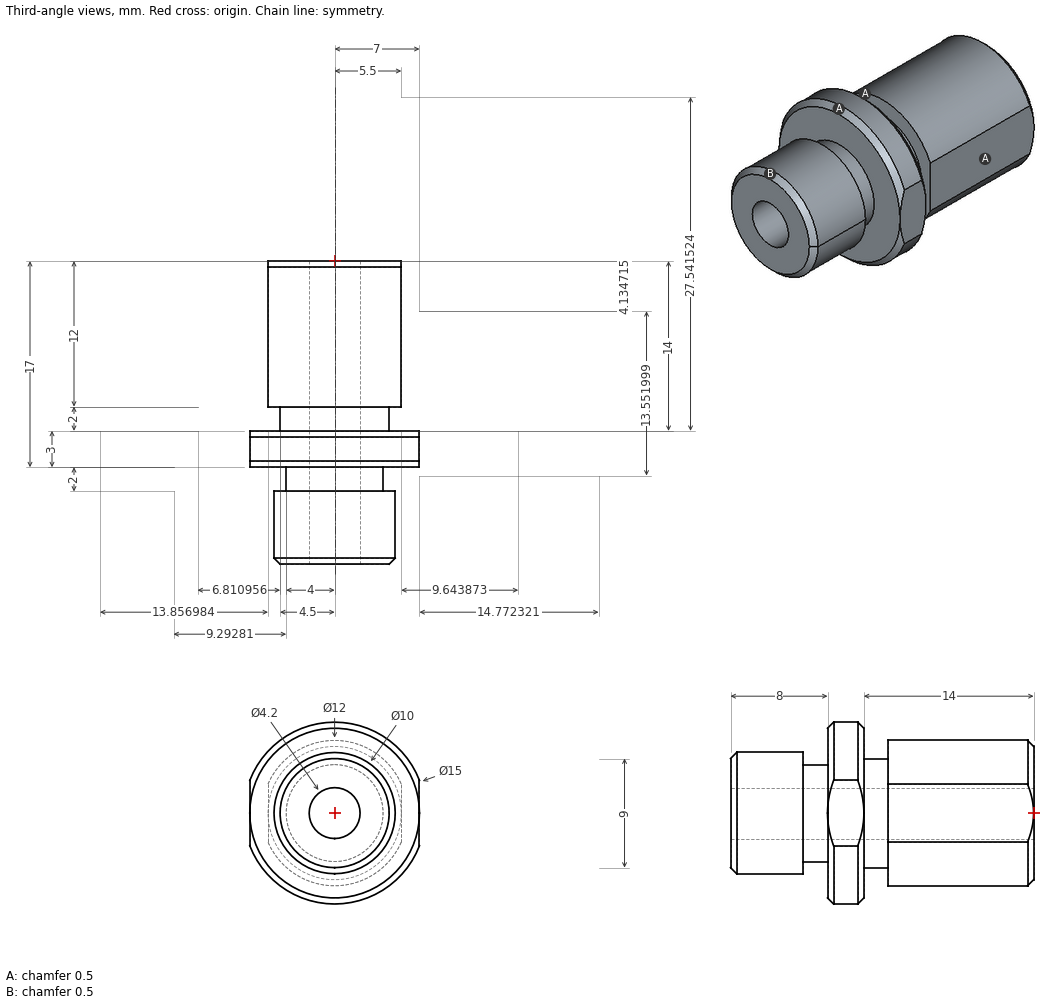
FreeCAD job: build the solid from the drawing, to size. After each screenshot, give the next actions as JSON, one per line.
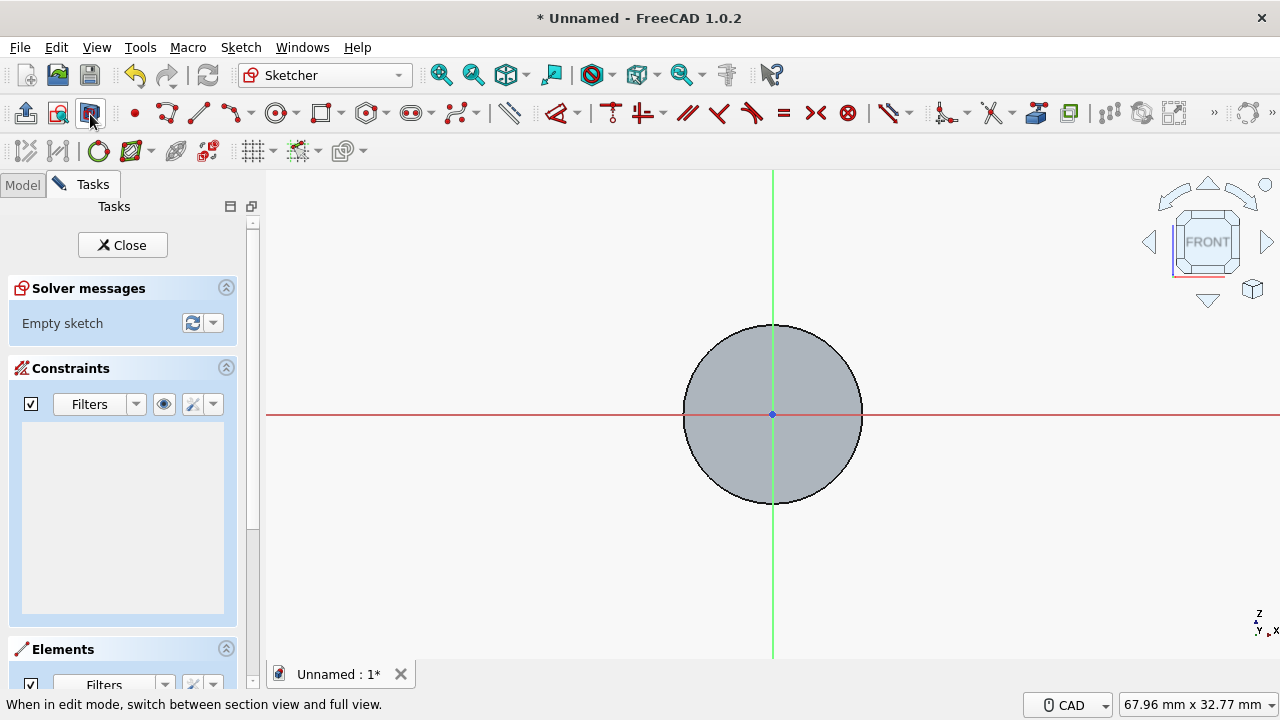
{"action": "scroll", "coordinate": [790, 414], "scroll_direction": "up", "scroll_amount": 8}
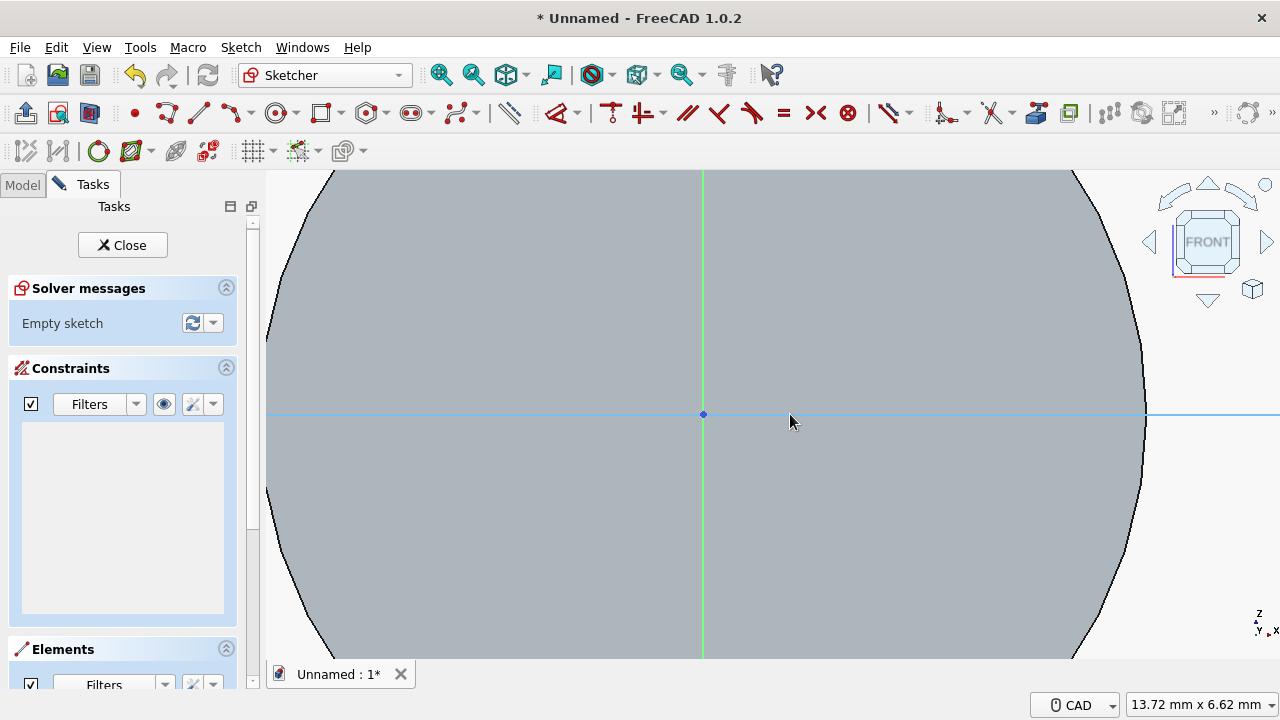
{"action": "left_click", "coordinate": [276, 114]}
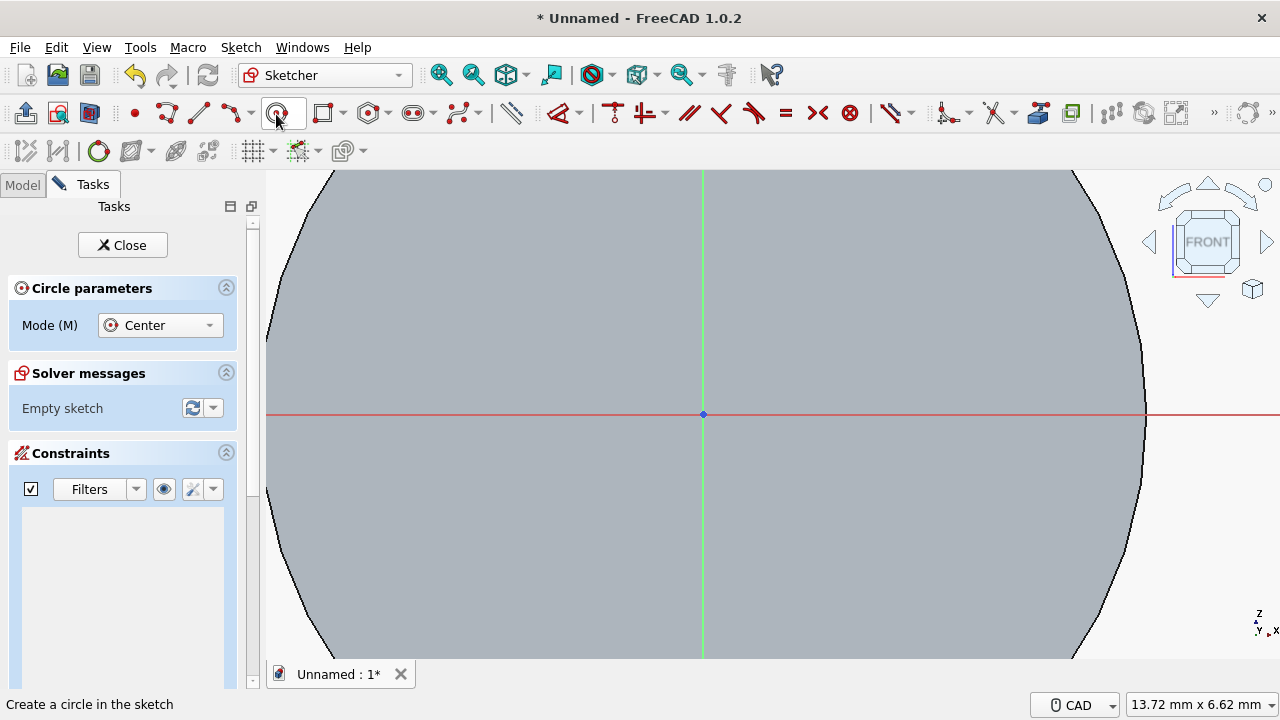
{"action": "left_click", "coordinate": [703, 414]}
{"action": "left_click", "coordinate": [813, 305]}
{"action": "key", "text": "Escape"}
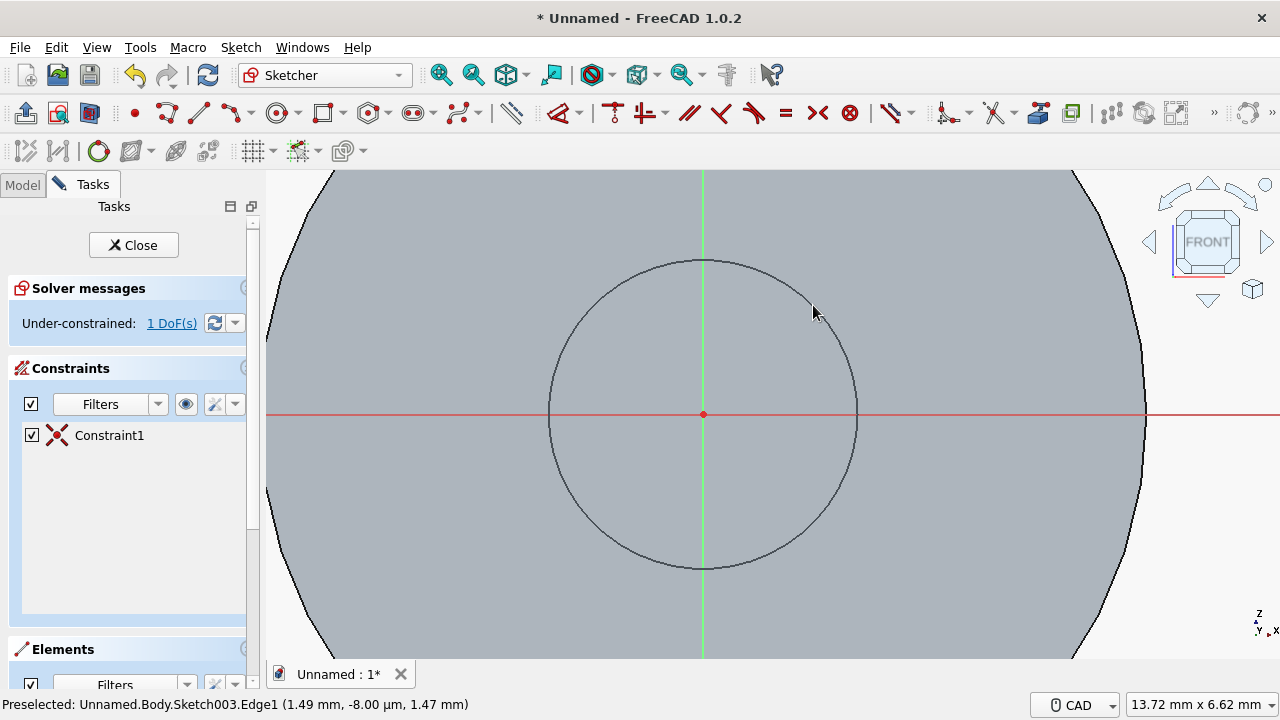
{"action": "key", "text": "d"}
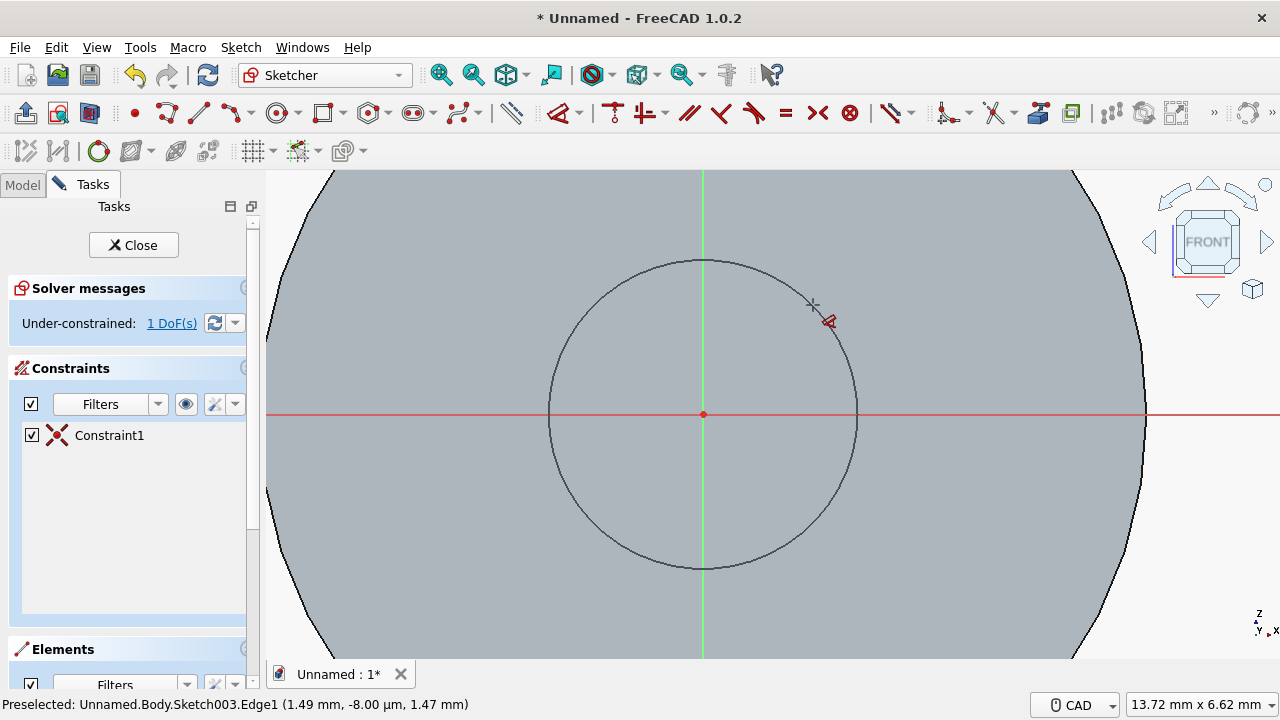
{"action": "left_click", "coordinate": [812, 305]}
{"action": "left_click", "coordinate": [835, 282]}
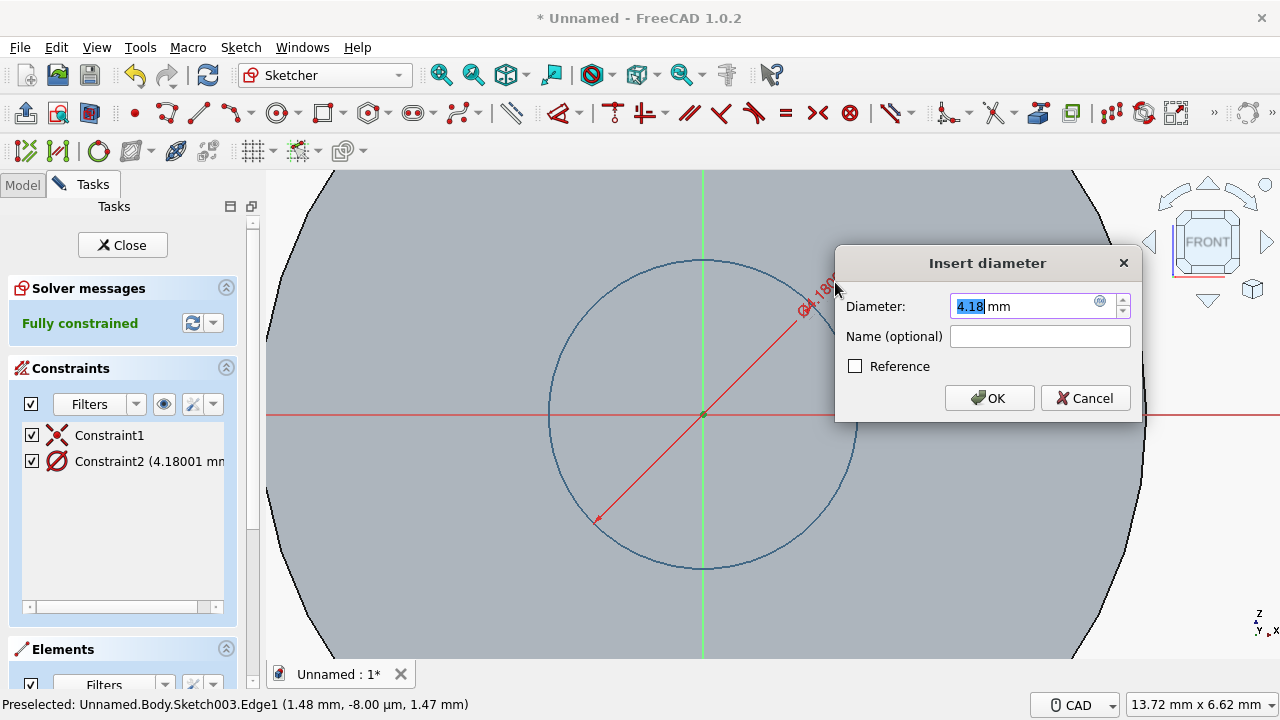
{"action": "type", "text": "4.2"}
{"action": "key", "text": "Return"}
{"action": "key", "text": "Escape"}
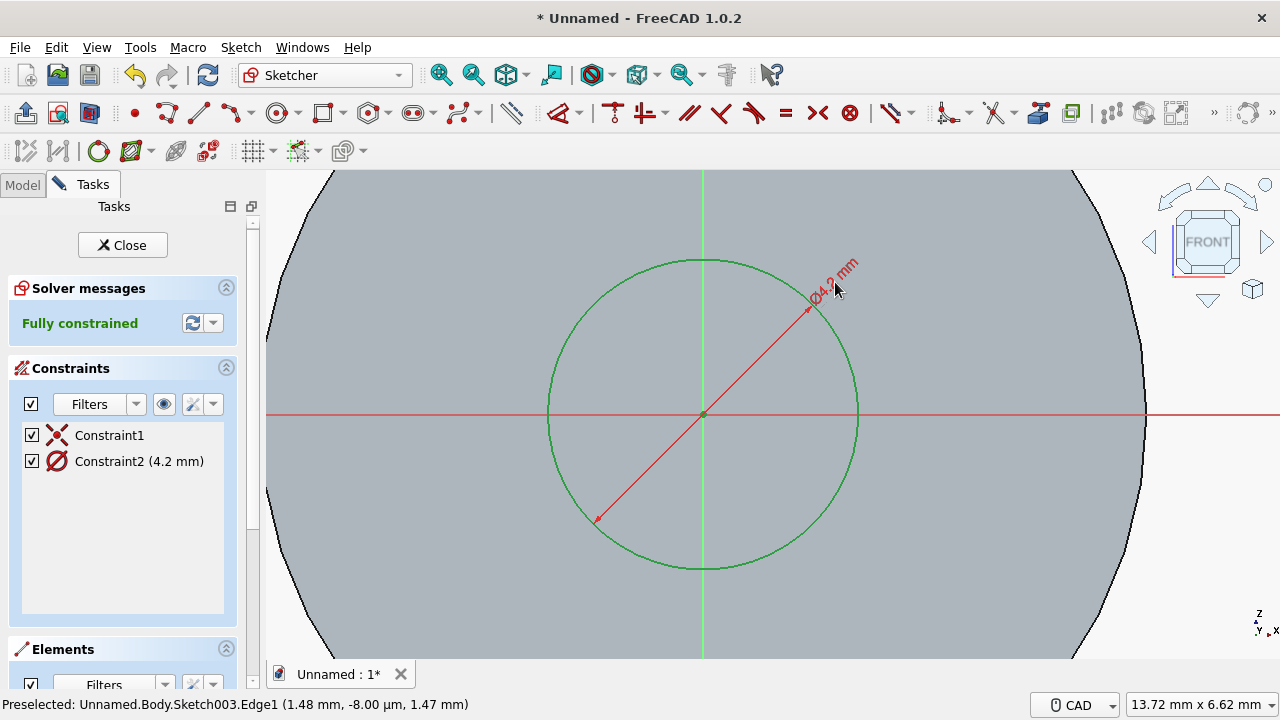
{"action": "left_click", "coordinate": [123, 245]}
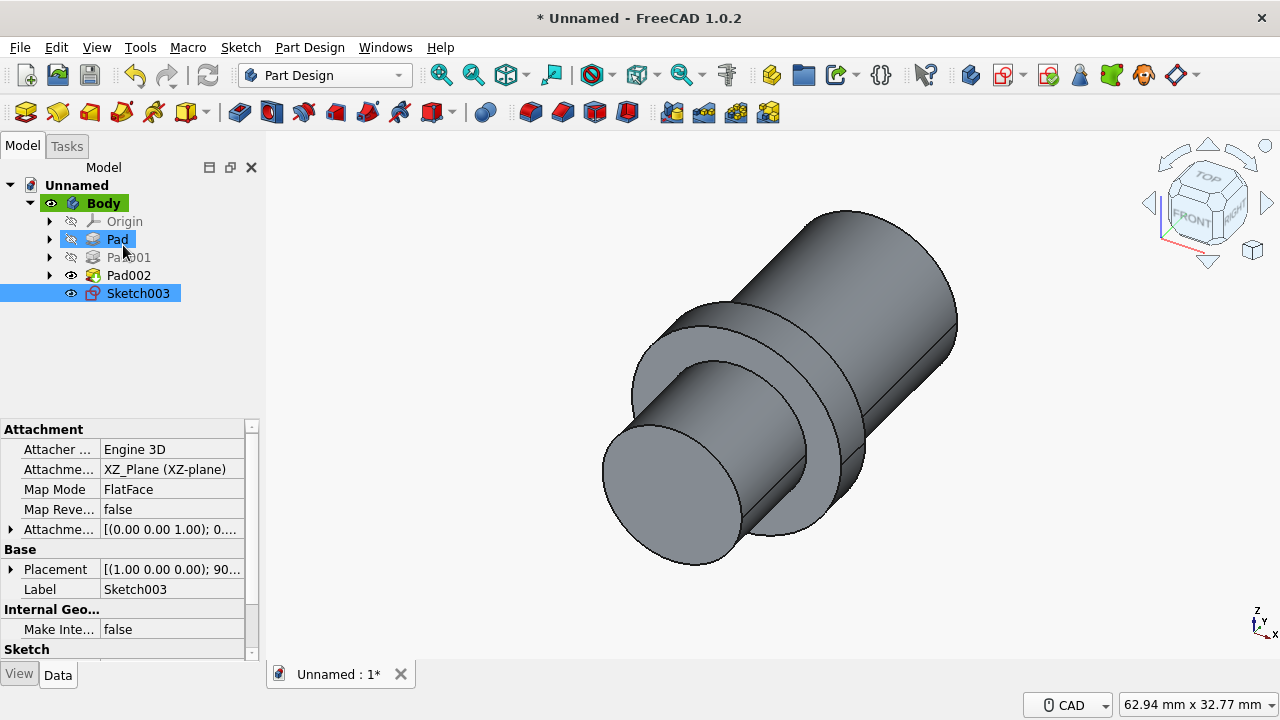
{"action": "left_click", "coordinate": [240, 112]}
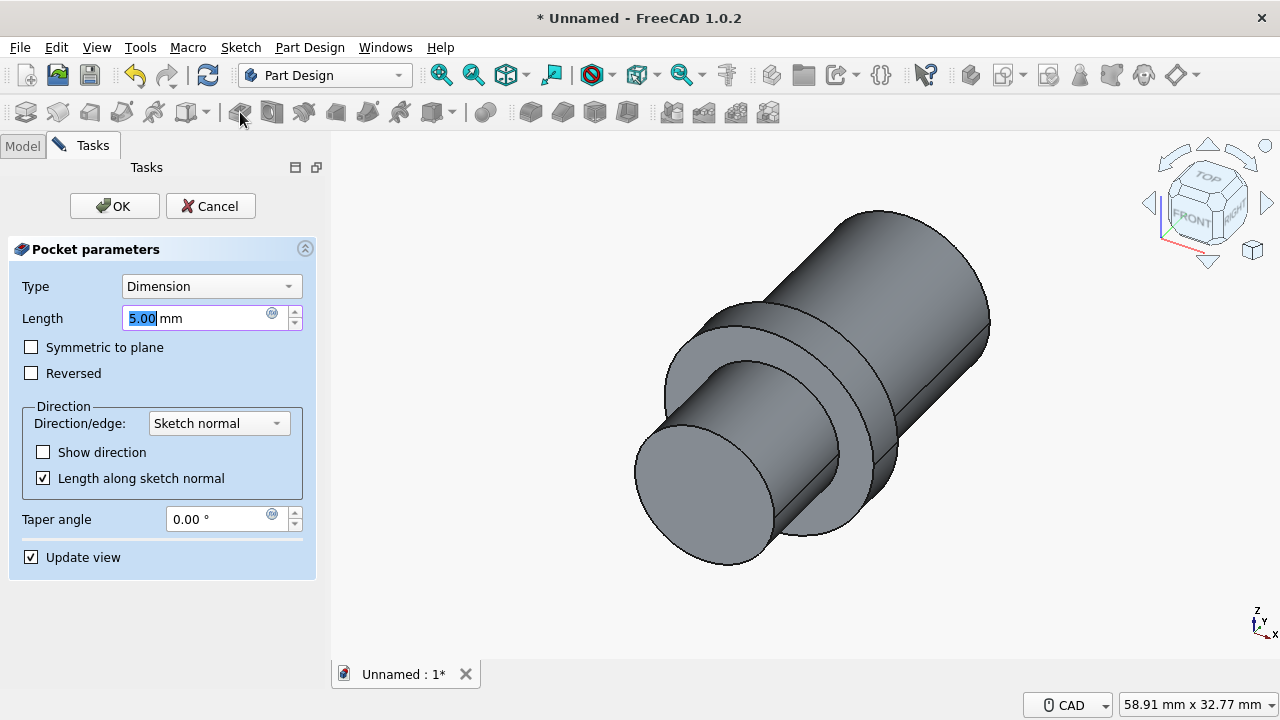
{"action": "left_click", "coordinate": [212, 286]}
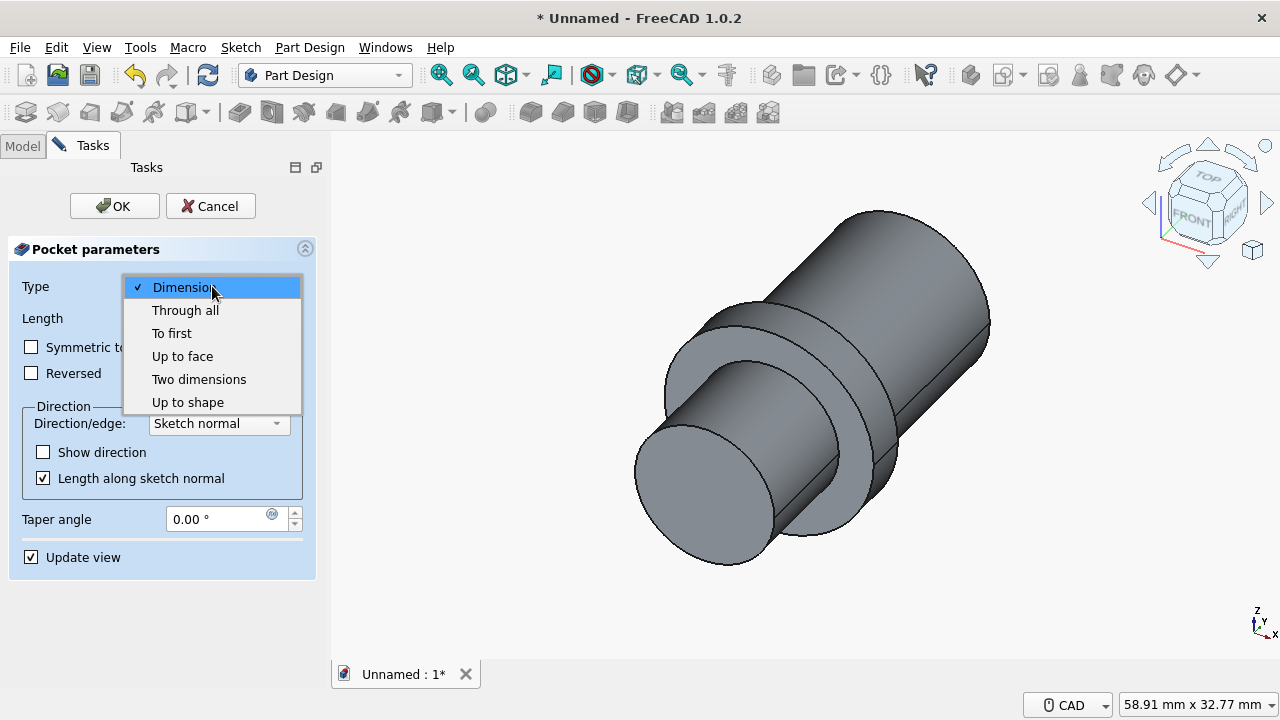
{"action": "left_click", "coordinate": [212, 310]}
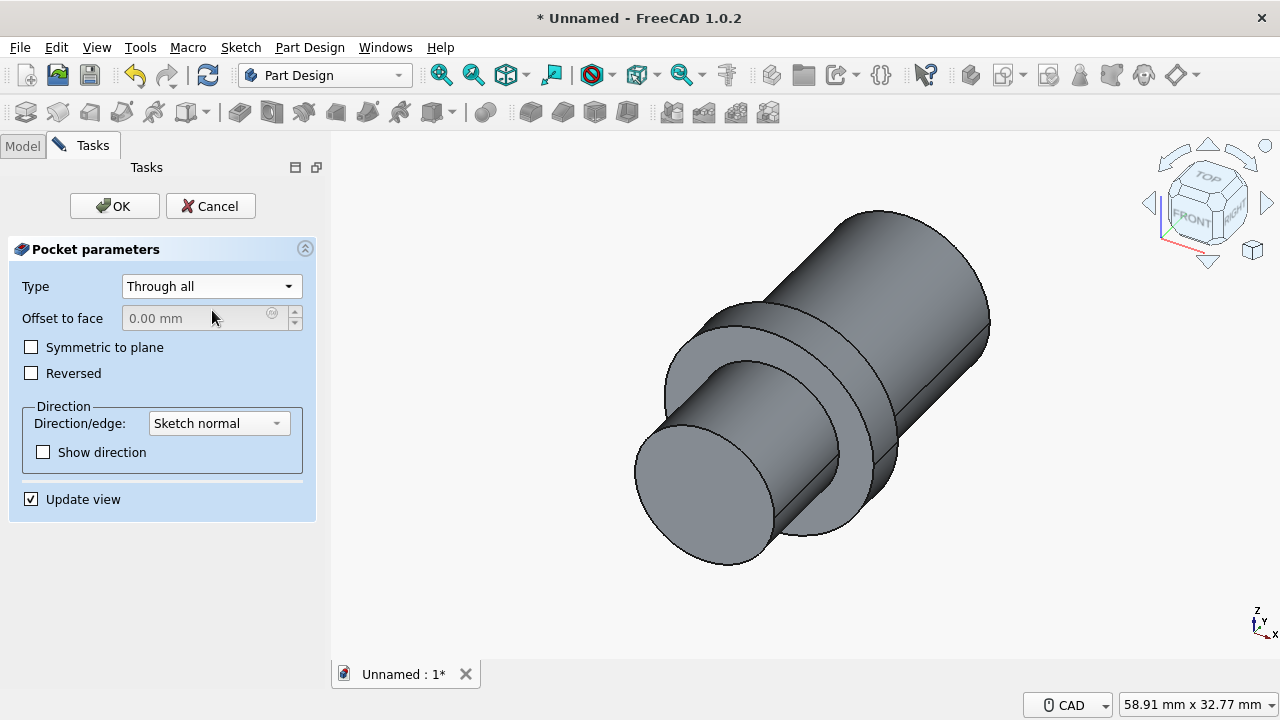
{"action": "left_click", "coordinate": [30, 373]}